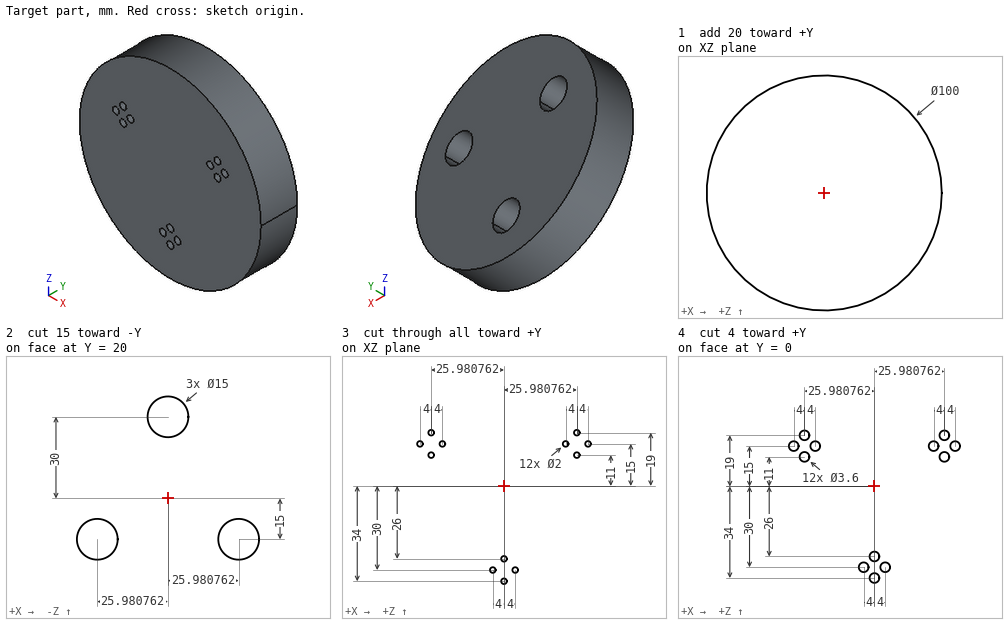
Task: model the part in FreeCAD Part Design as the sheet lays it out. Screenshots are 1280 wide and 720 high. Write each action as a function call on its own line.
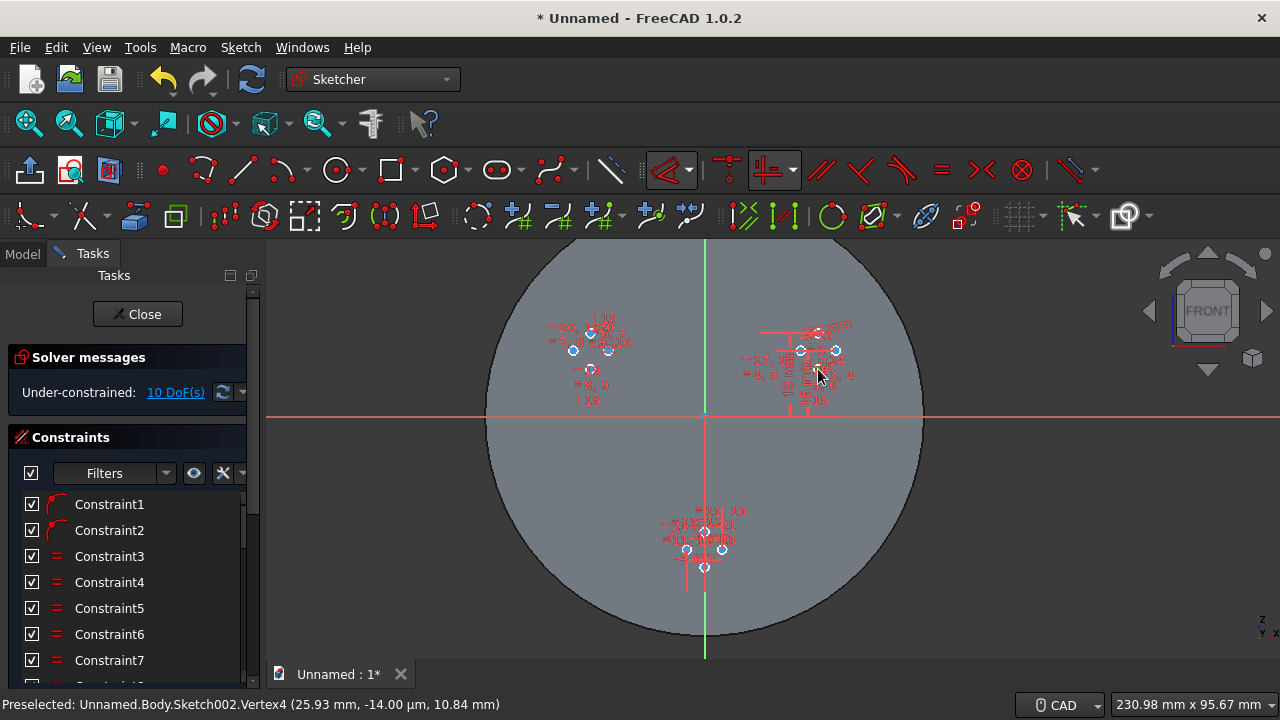
click(692, 170)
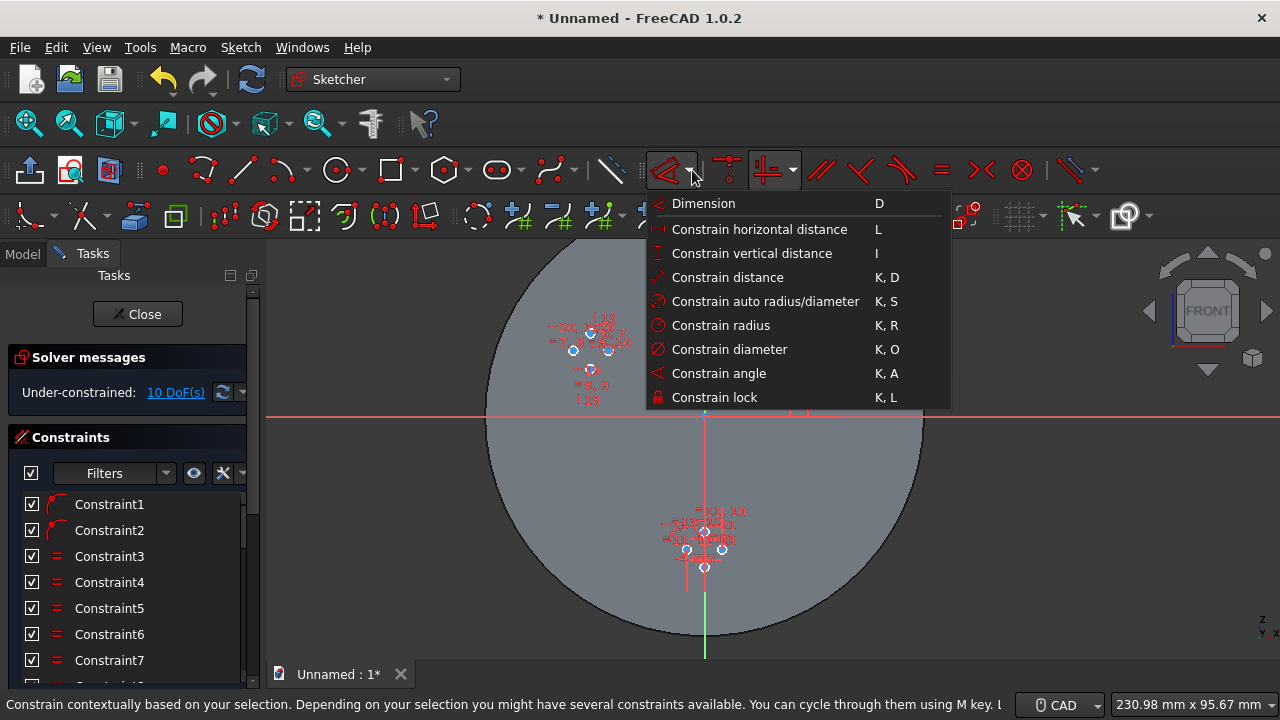
click(799, 253)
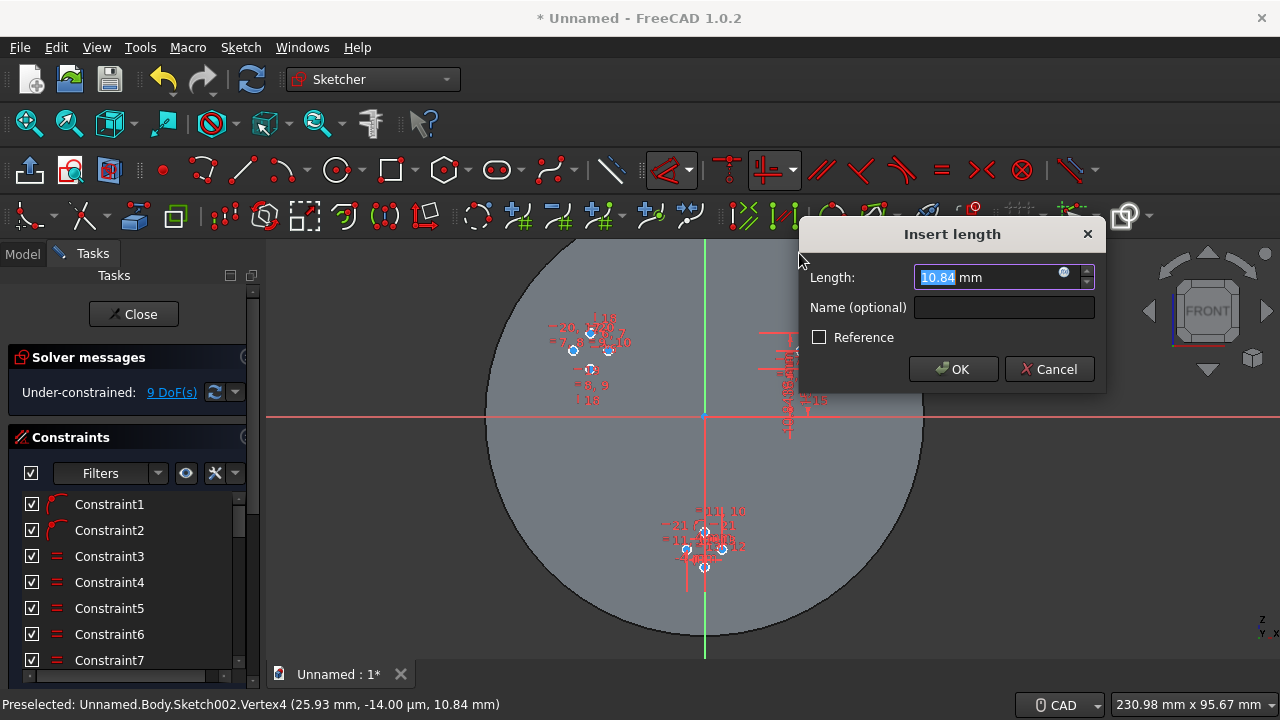
text(11)
key(Return)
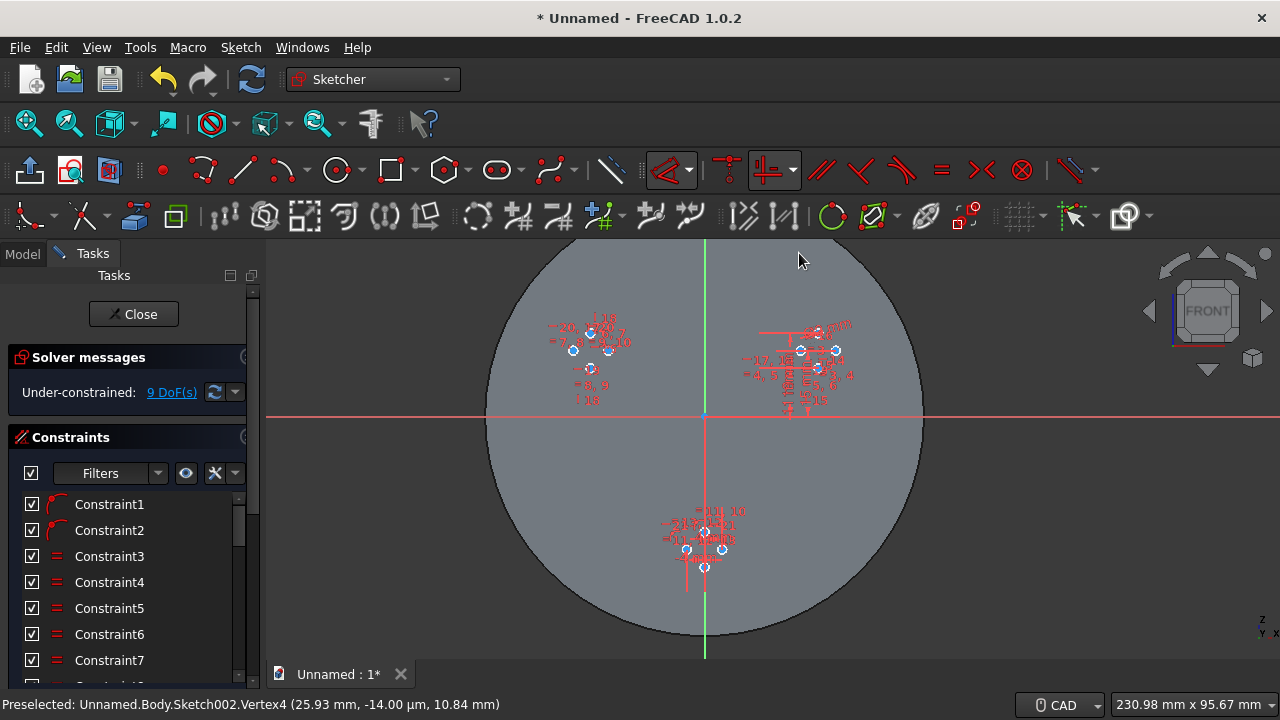
click(705, 532)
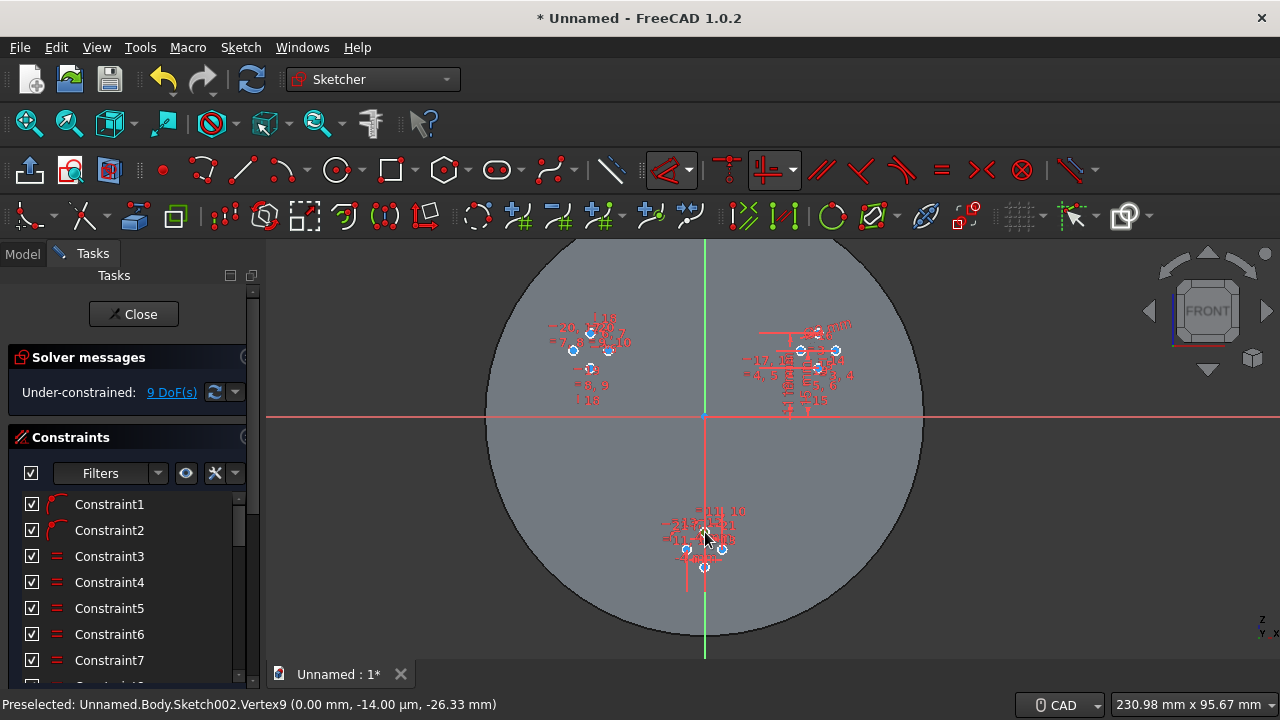
click(692, 170)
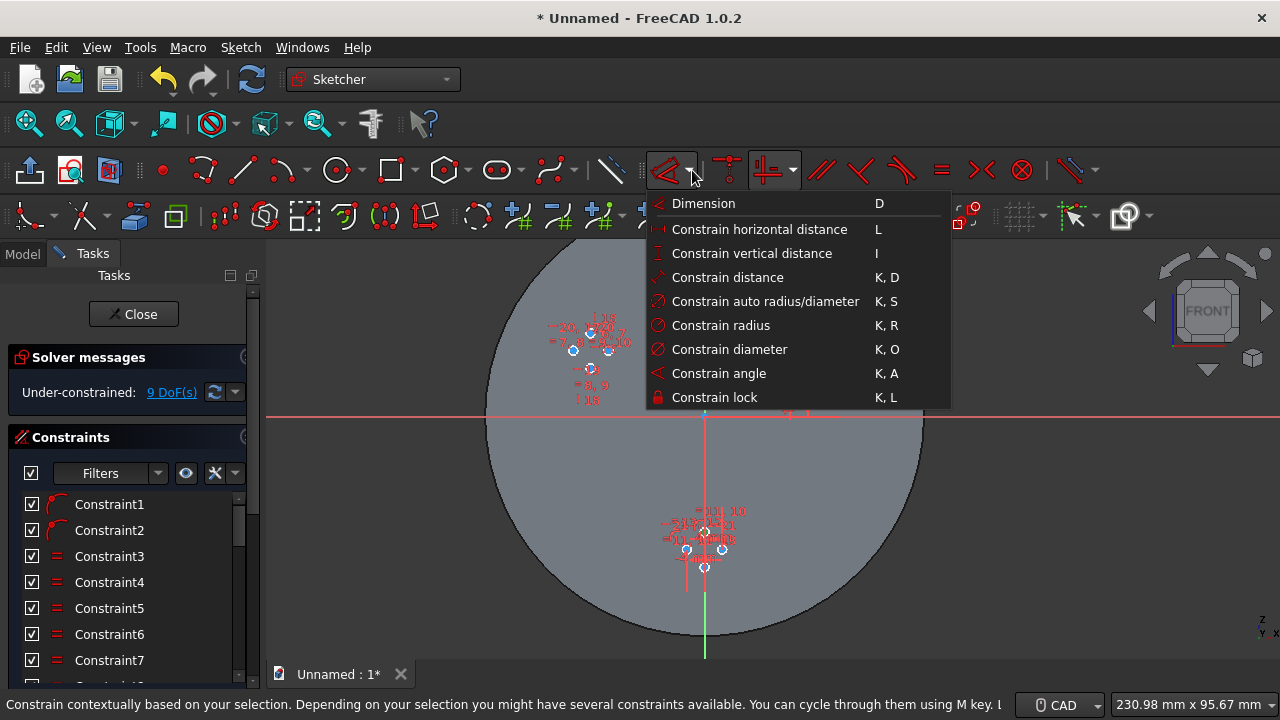
click(799, 253)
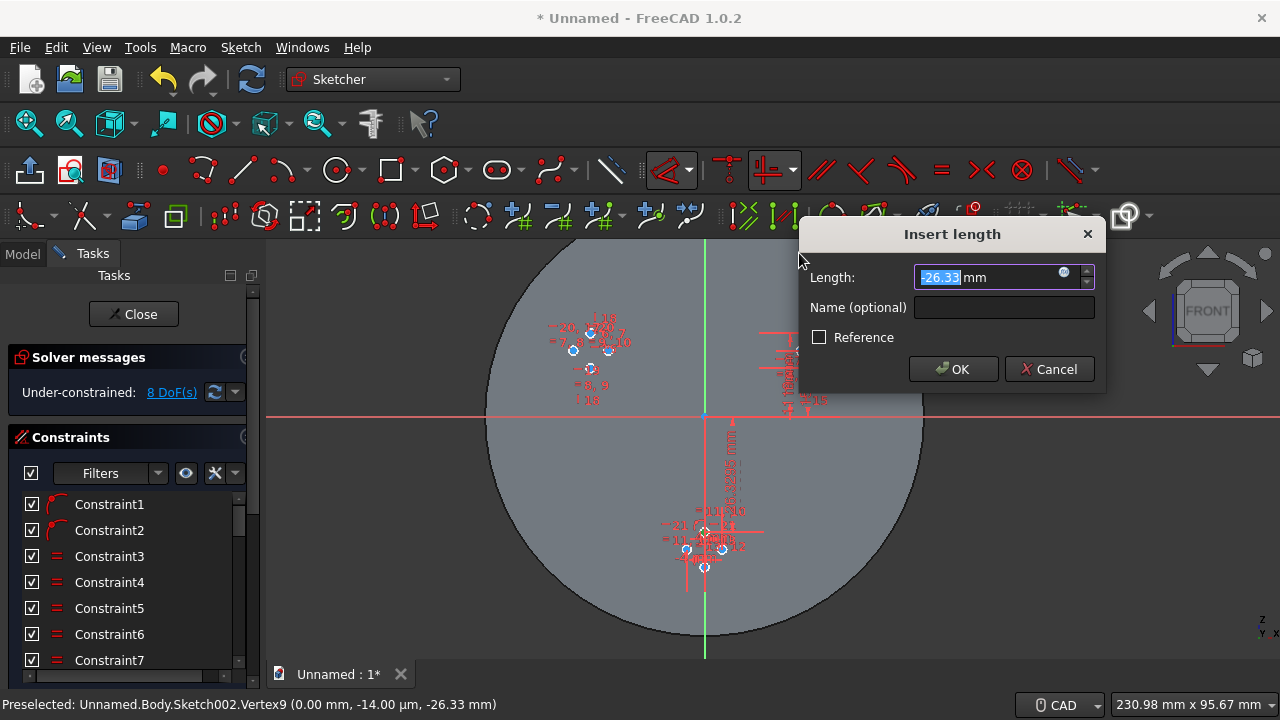
text(-26)
key(Return)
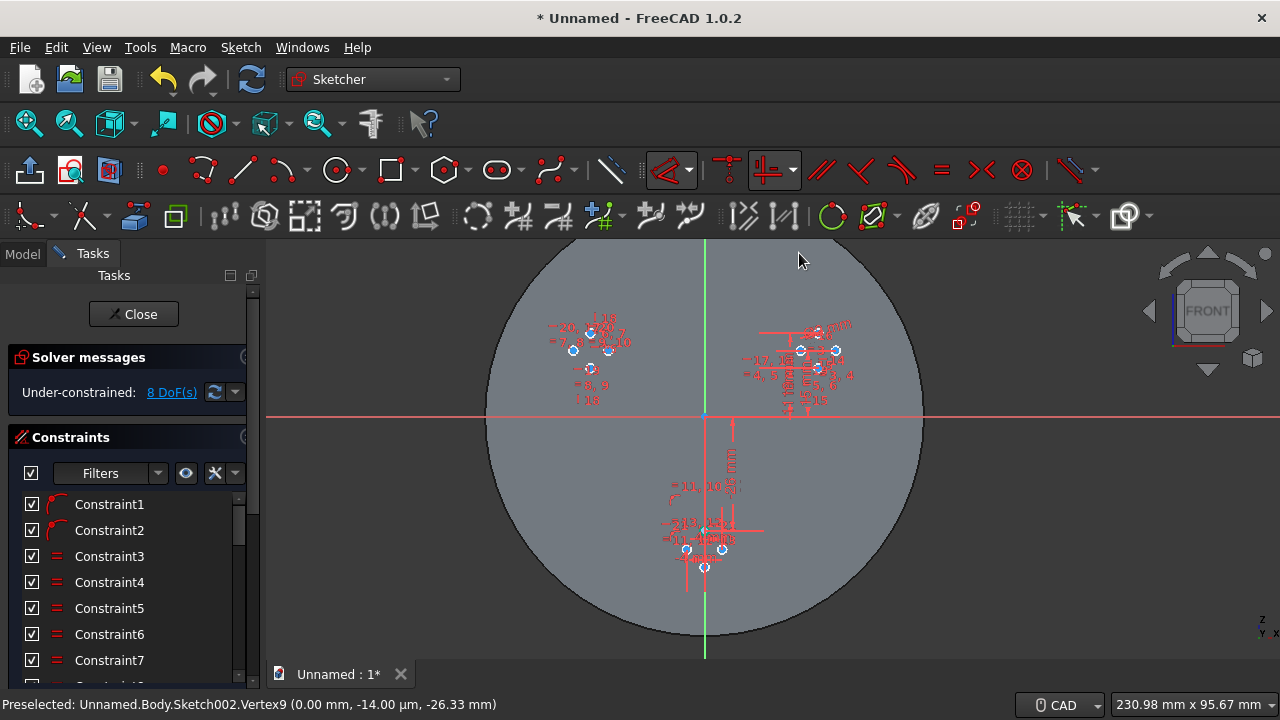
click(687, 550)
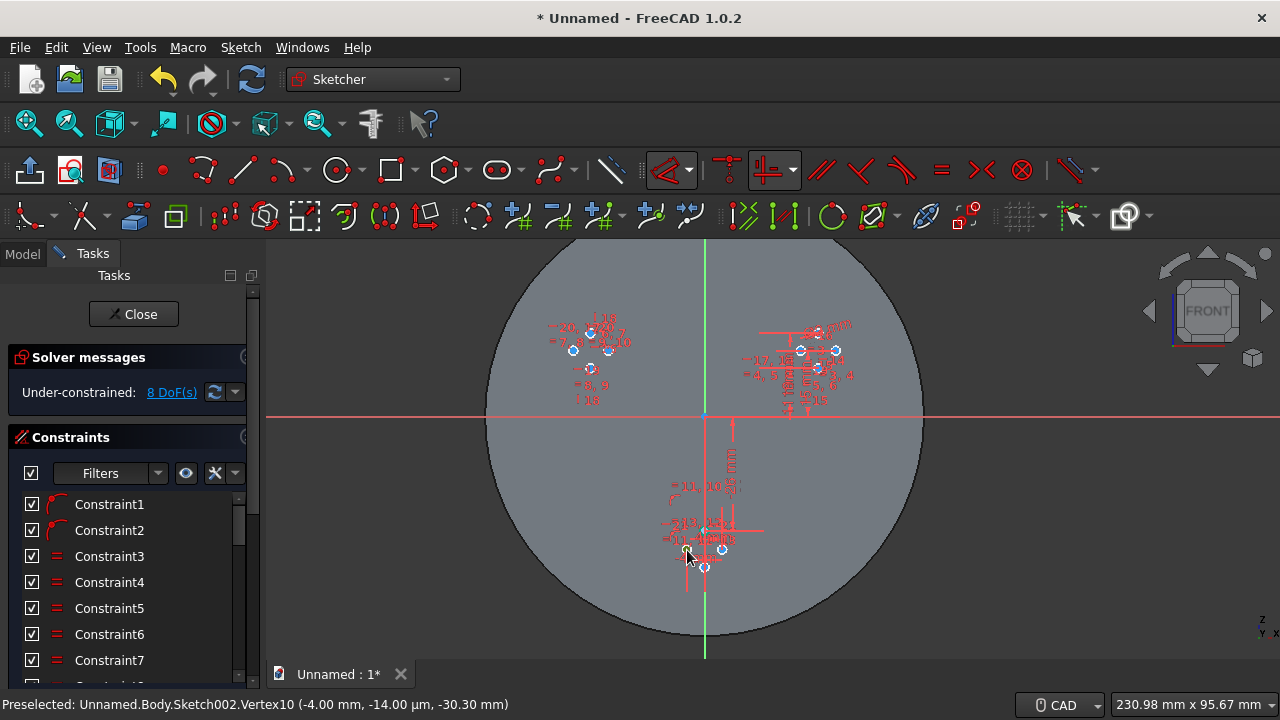
key(i)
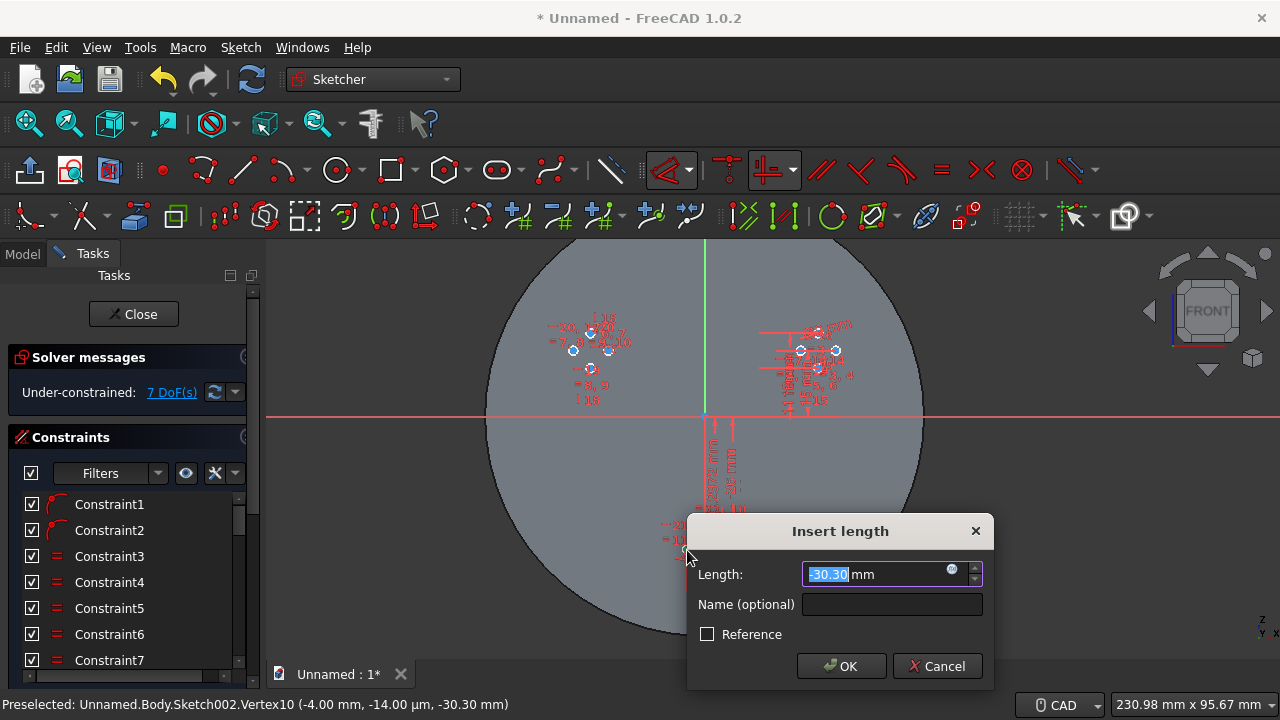
text(-30)
key(Return)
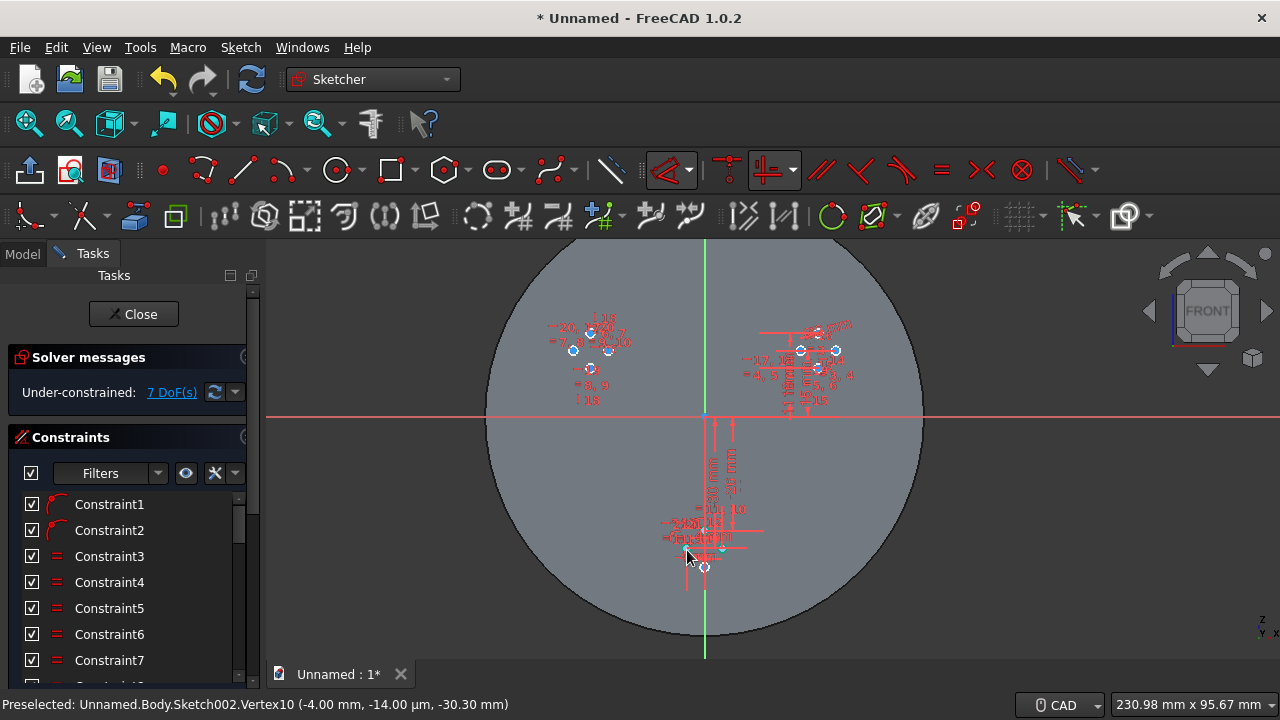
click(705, 567)